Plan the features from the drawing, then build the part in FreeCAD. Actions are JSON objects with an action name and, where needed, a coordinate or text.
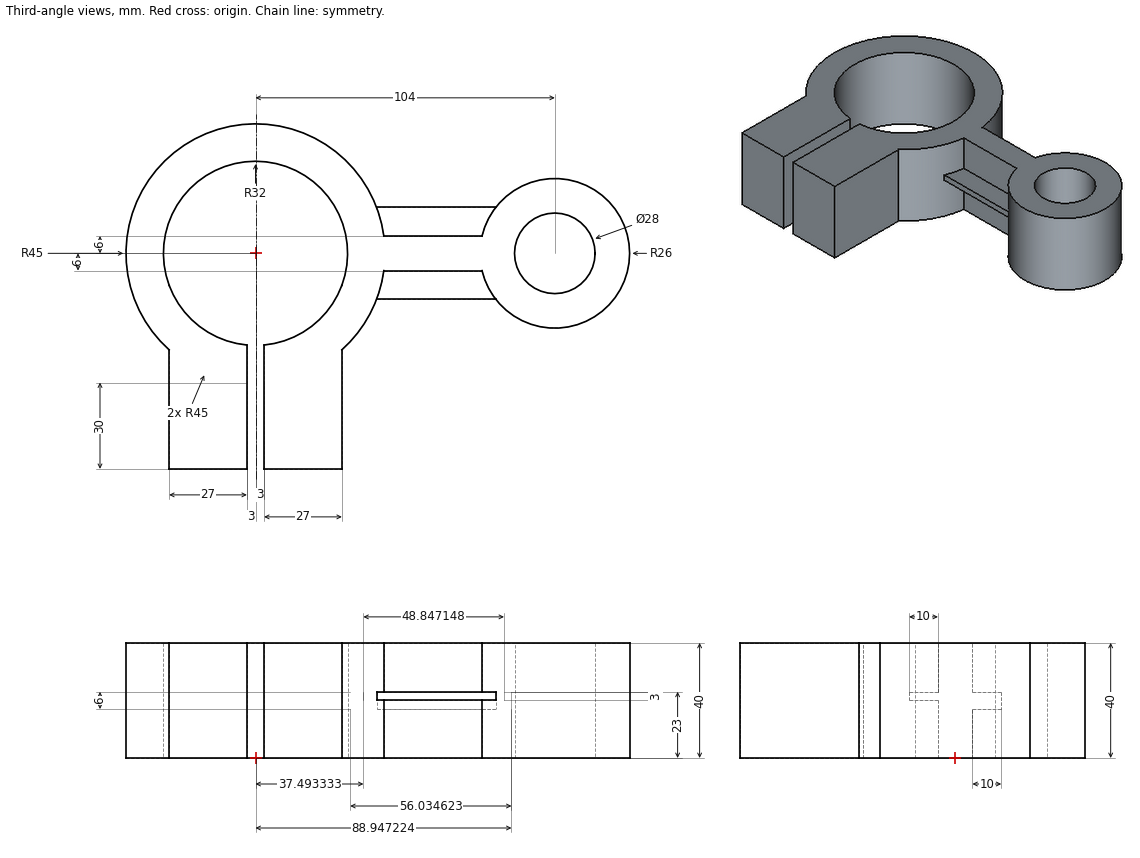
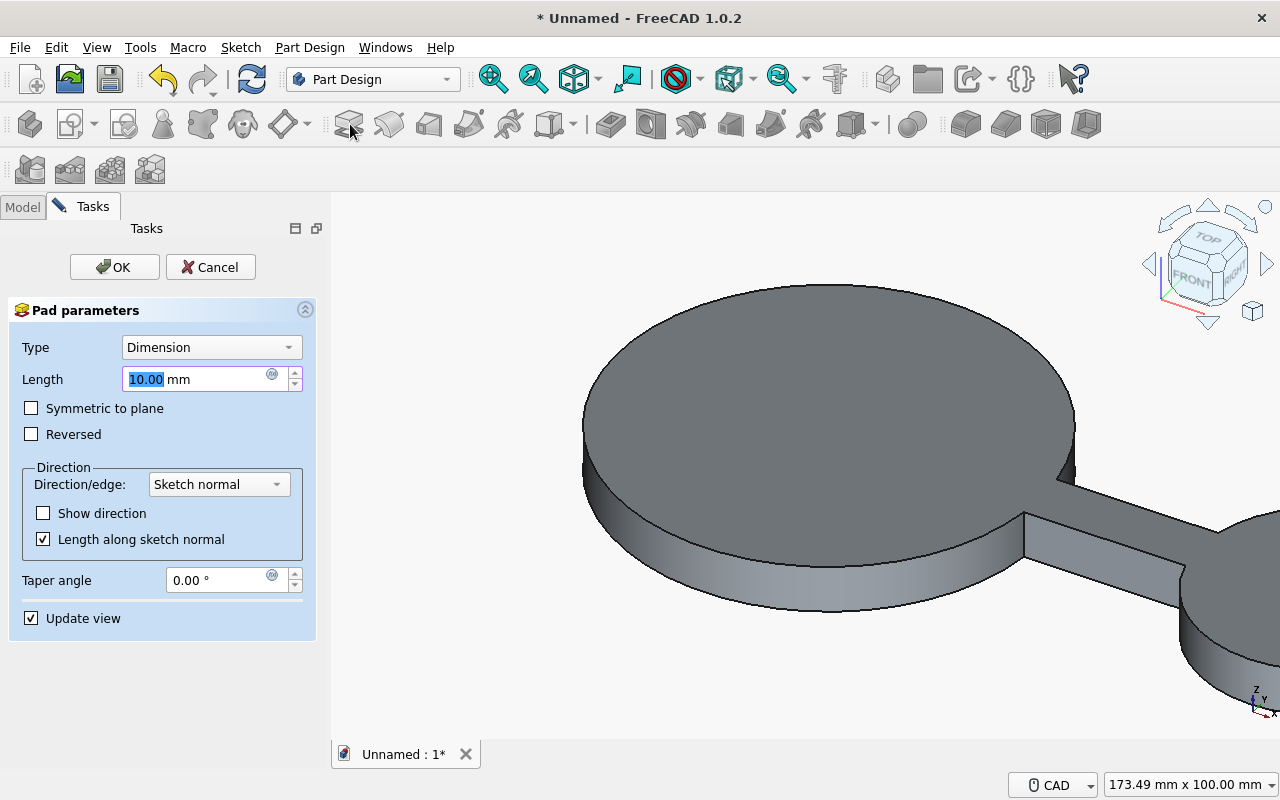
{"action": "type", "text": "40"}
{"action": "key", "text": "Tab"}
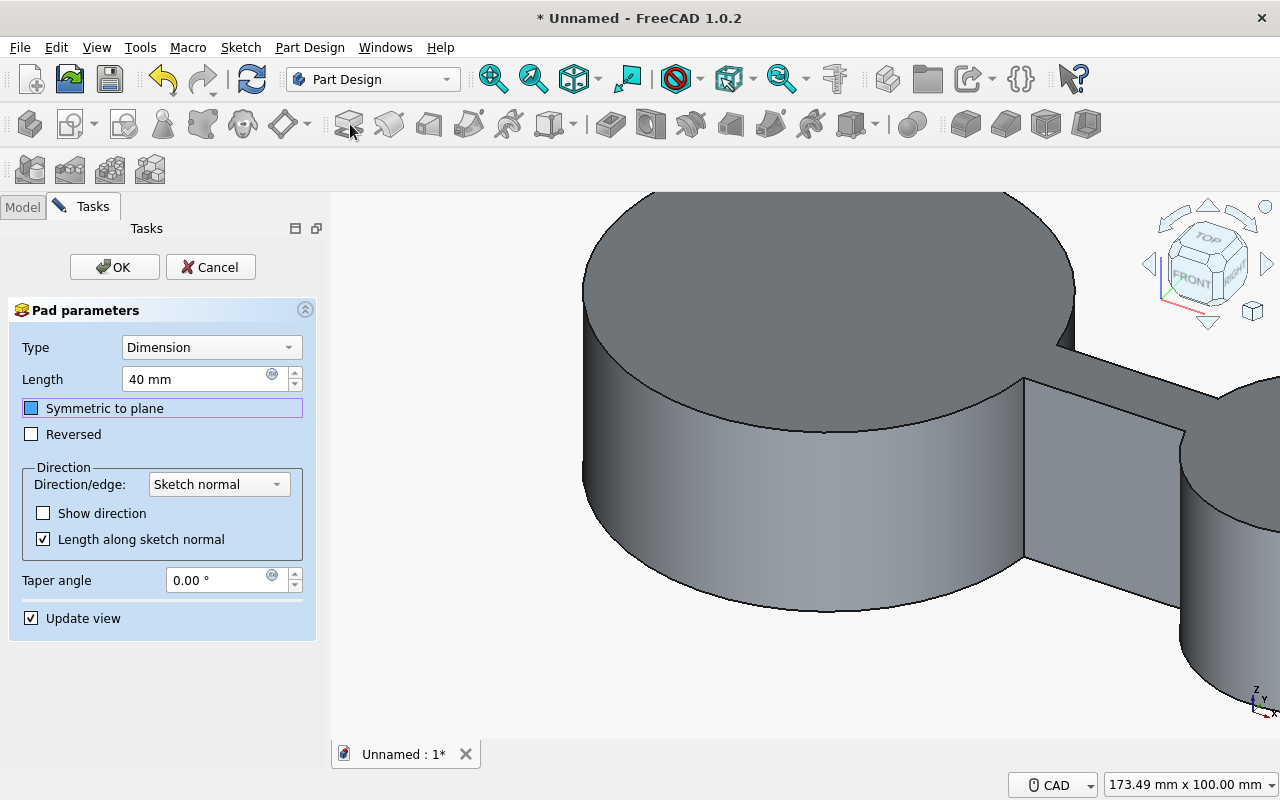
{"action": "left_click", "coordinate": [115, 267]}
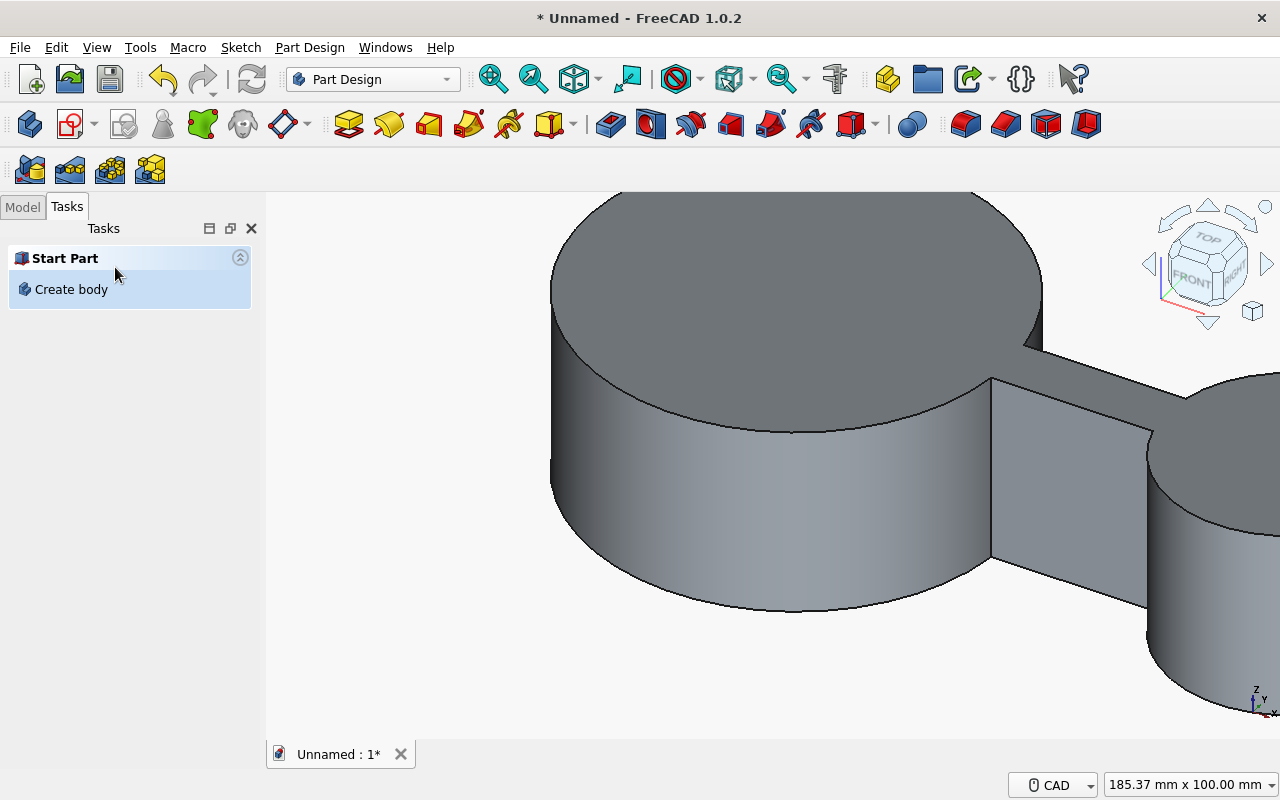
{"action": "key", "text": "v f"}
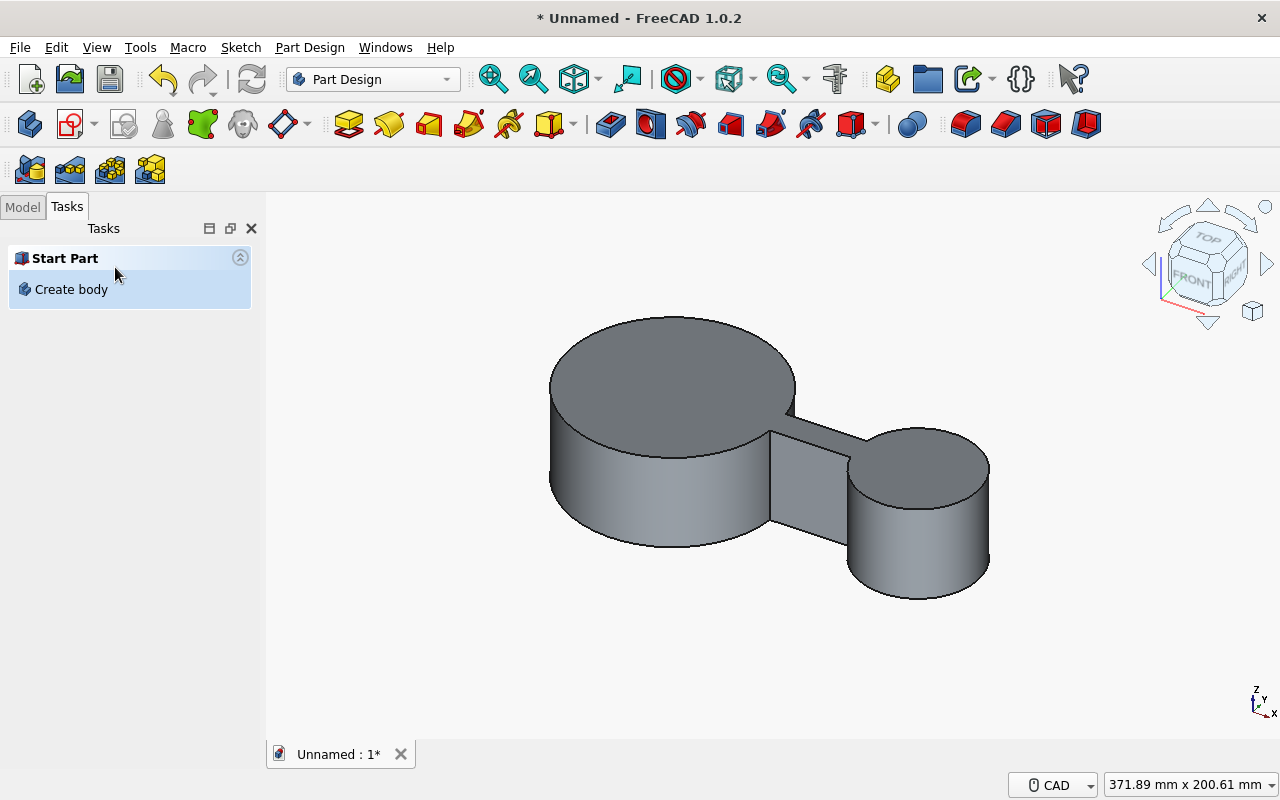
{"action": "left_click", "coordinate": [655, 381]}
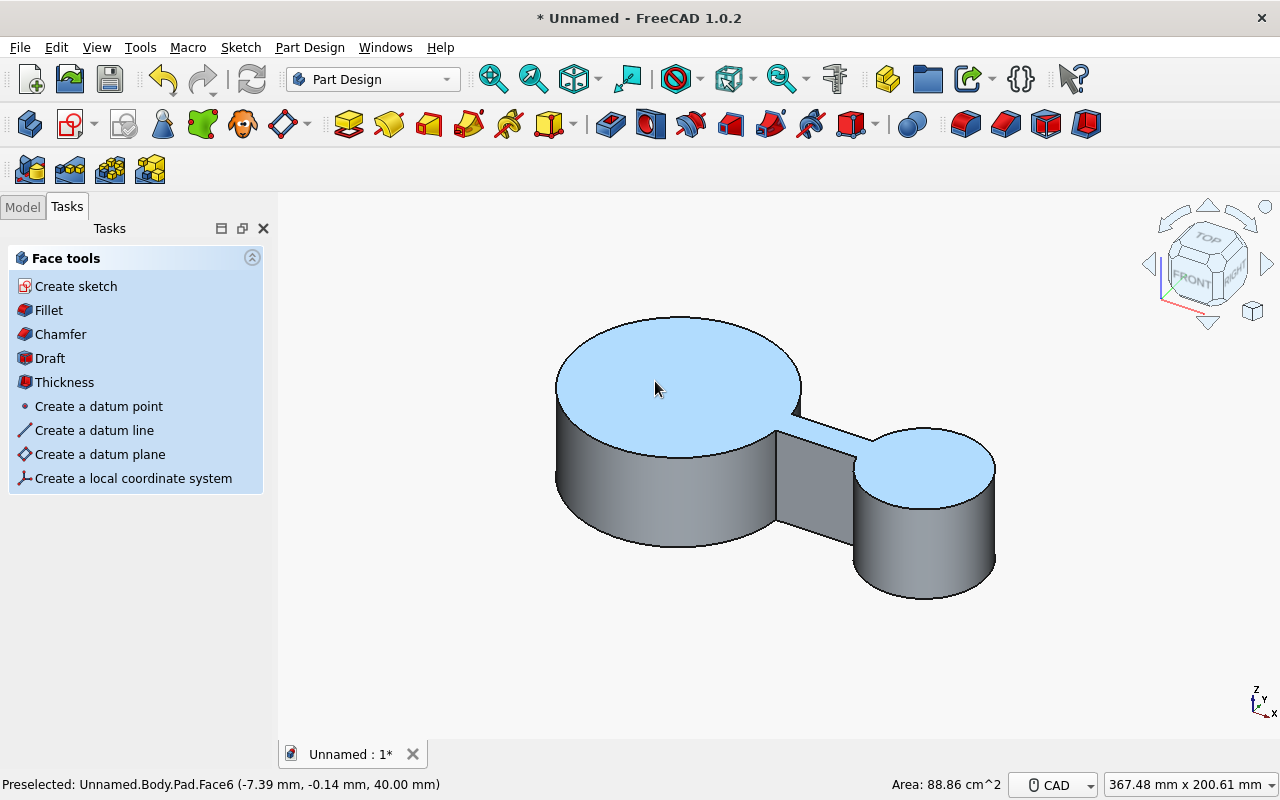
{"action": "left_click", "coordinate": [70, 124]}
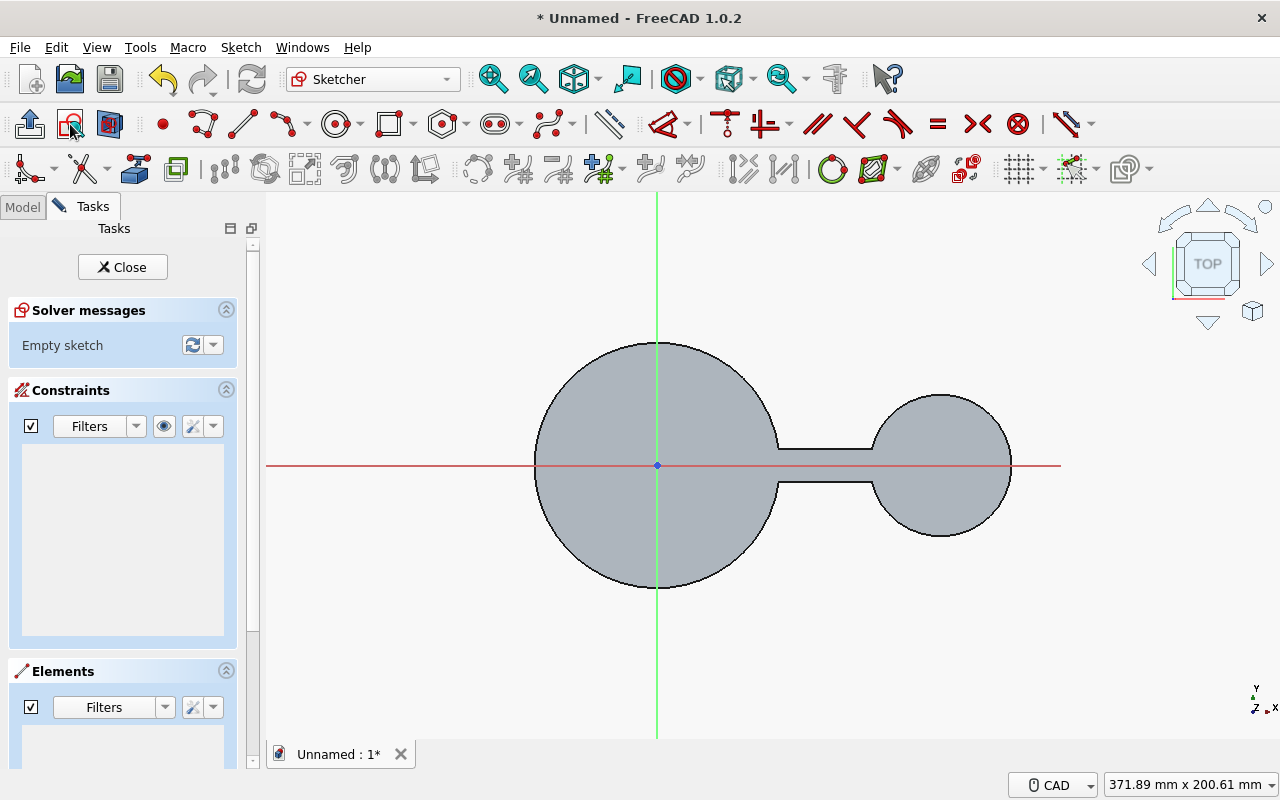
{"action": "scroll", "coordinate": [1000, 466], "scroll_direction": "up", "scroll_amount": 8}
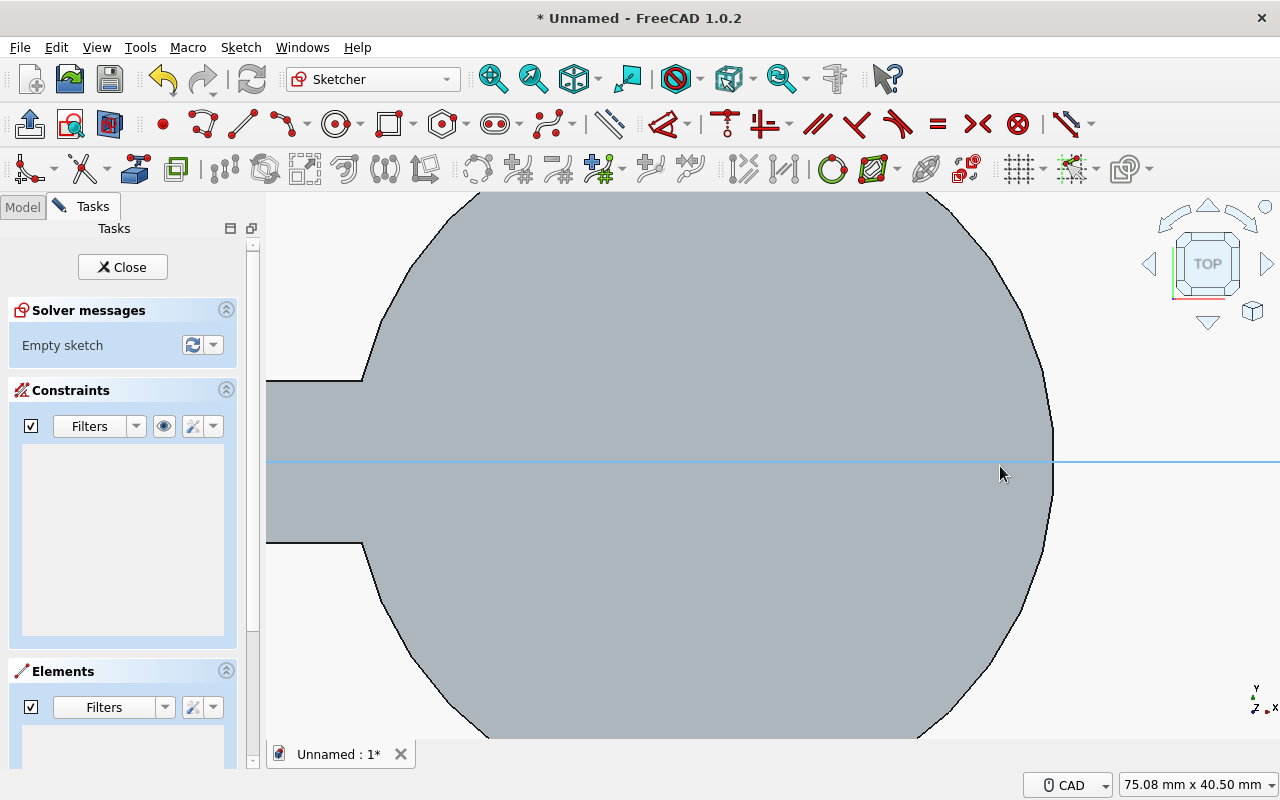
{"action": "key", "text": "g c"}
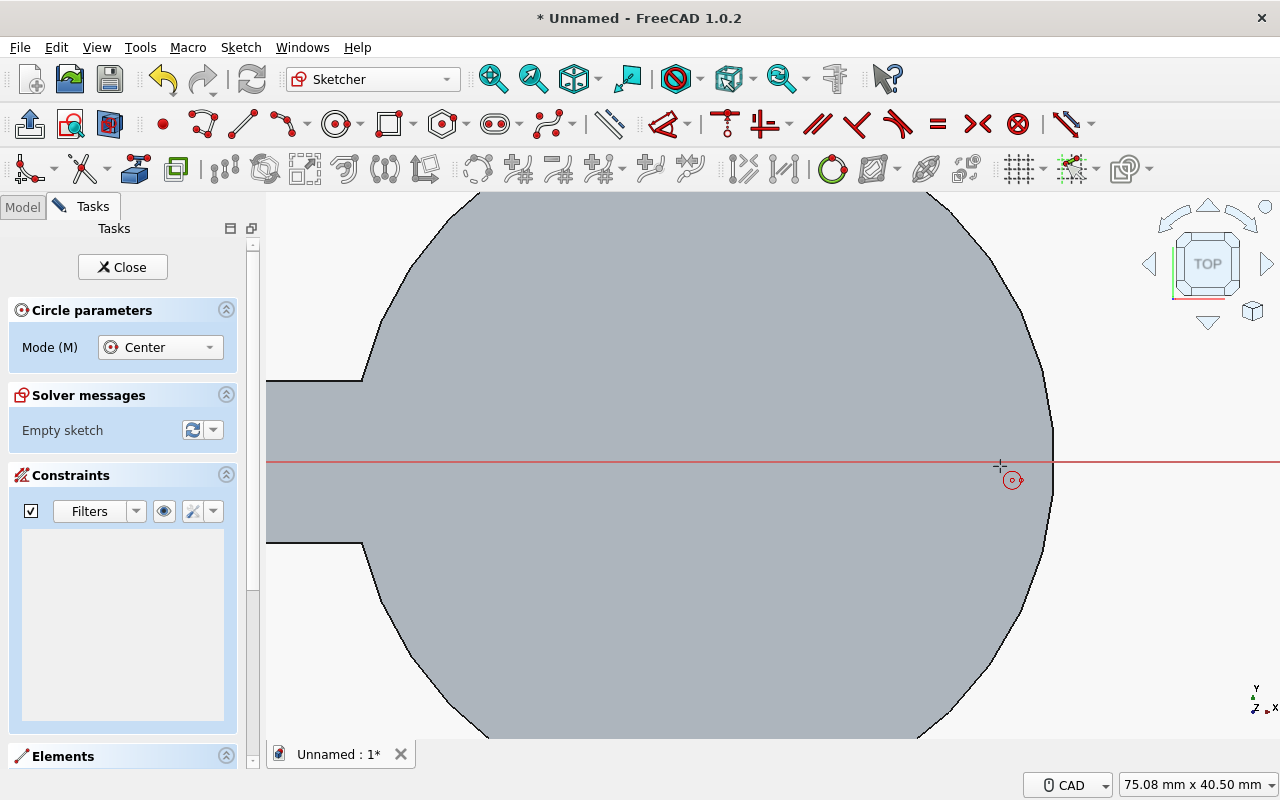
{"action": "left_click", "coordinate": [703, 462]}
{"action": "mouse_move", "coordinate": [837, 328]}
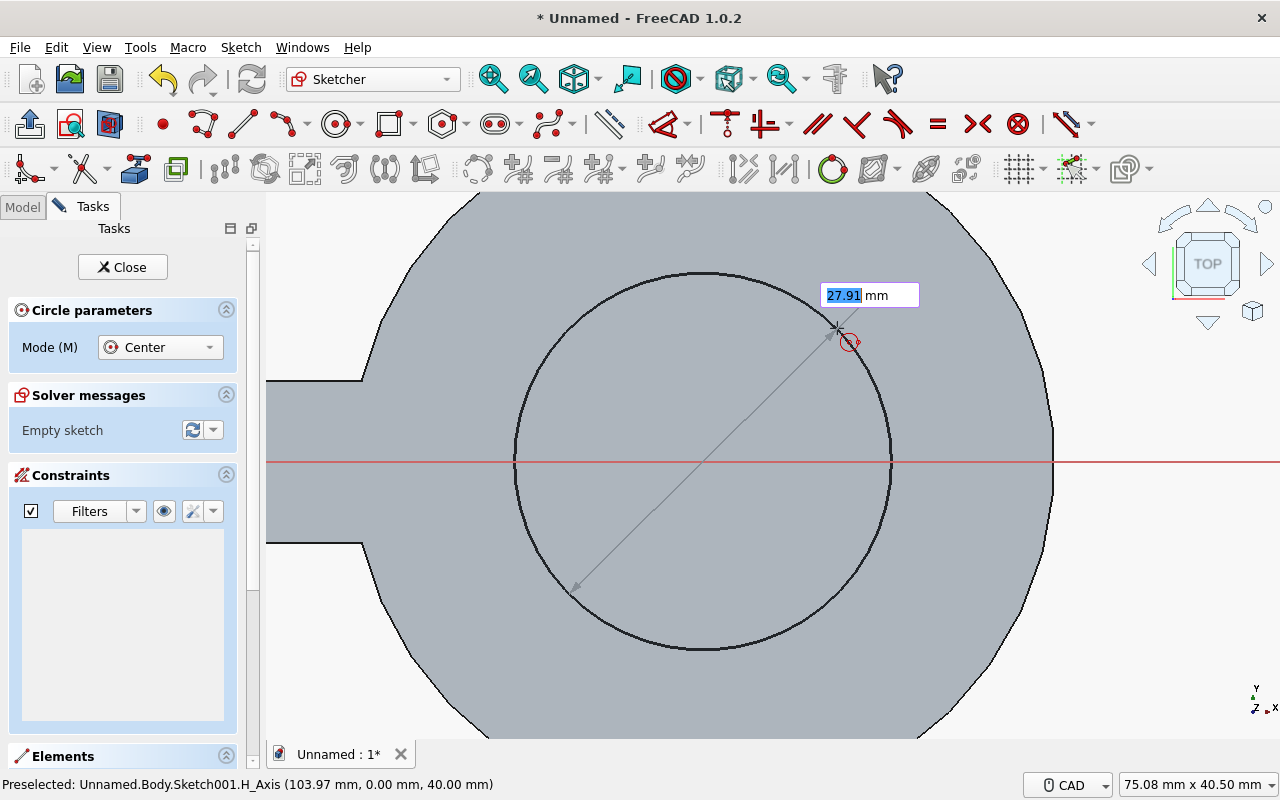
{"action": "type", "text": "28"}
{"action": "key", "text": "Return"}
{"action": "key", "text": "Escape"}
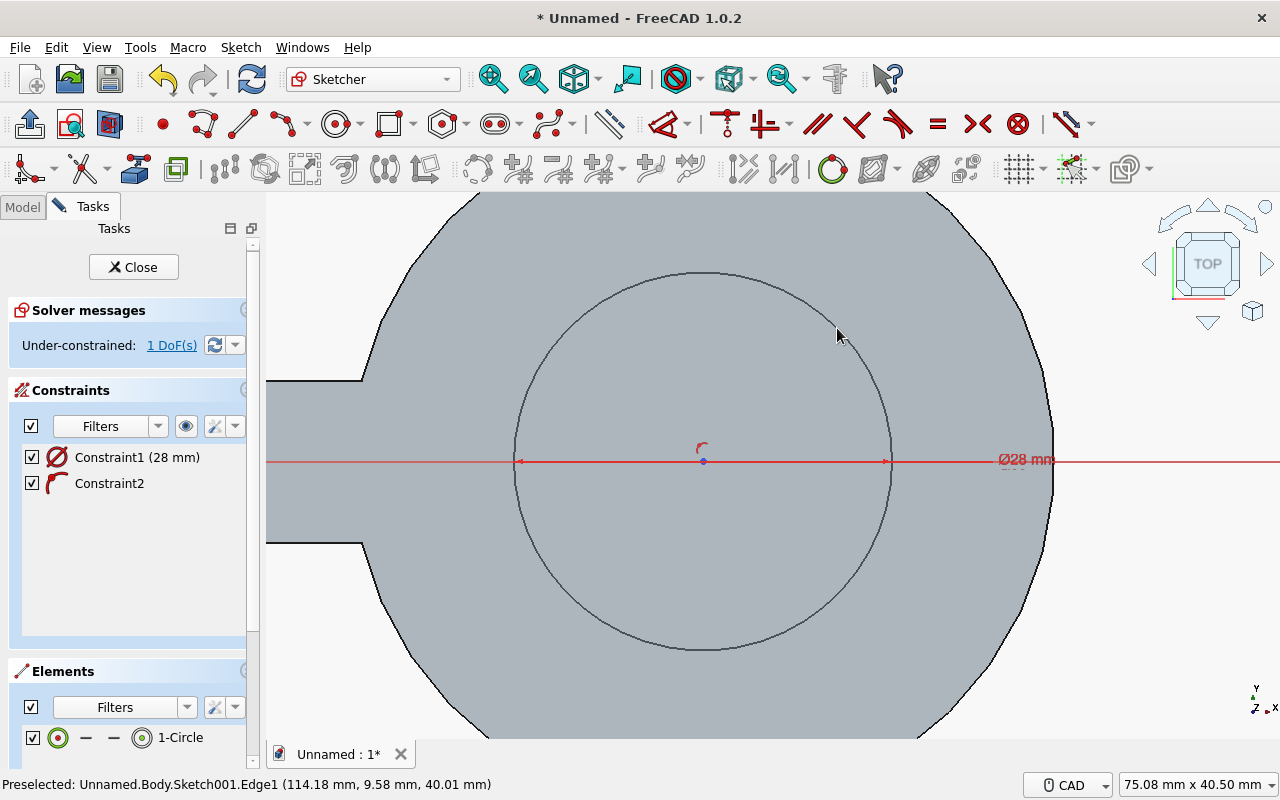
{"action": "key", "text": "d"}